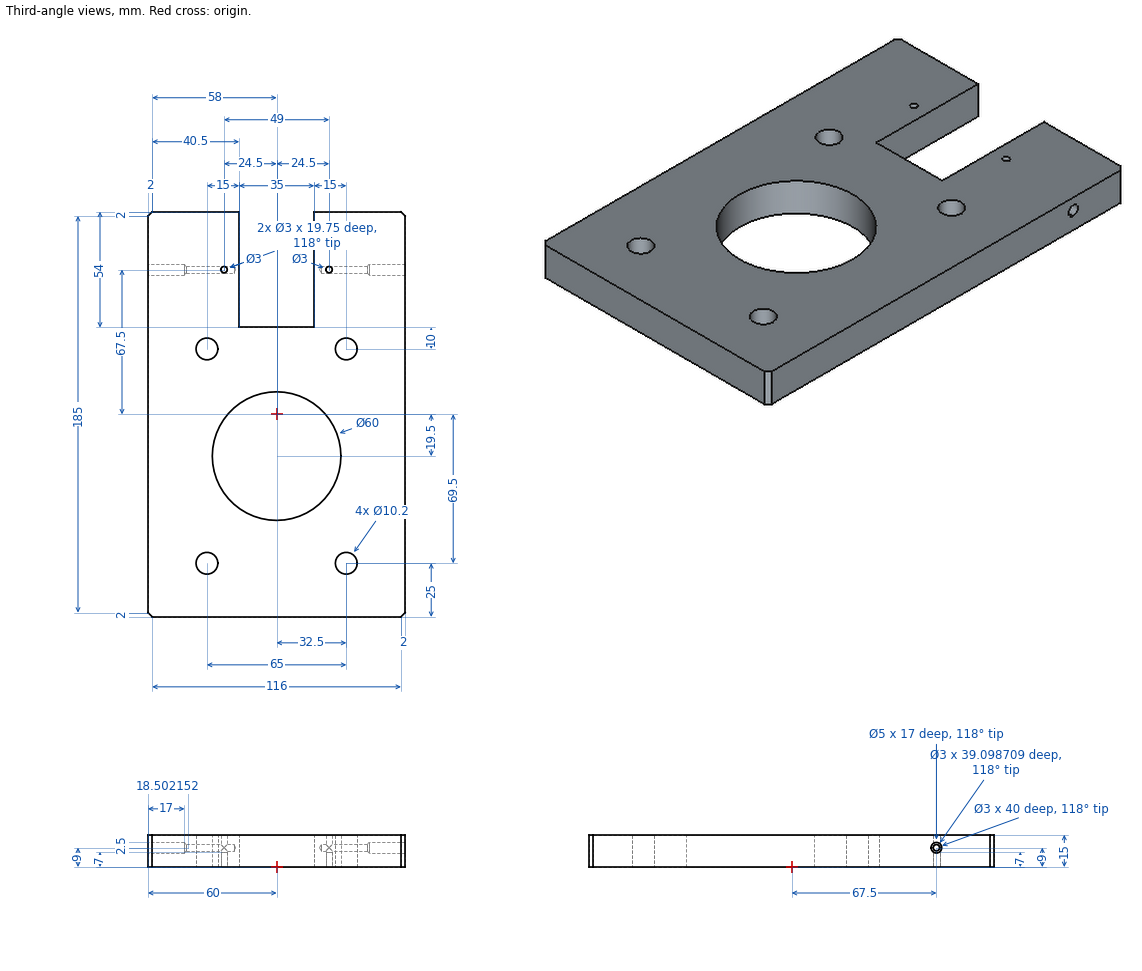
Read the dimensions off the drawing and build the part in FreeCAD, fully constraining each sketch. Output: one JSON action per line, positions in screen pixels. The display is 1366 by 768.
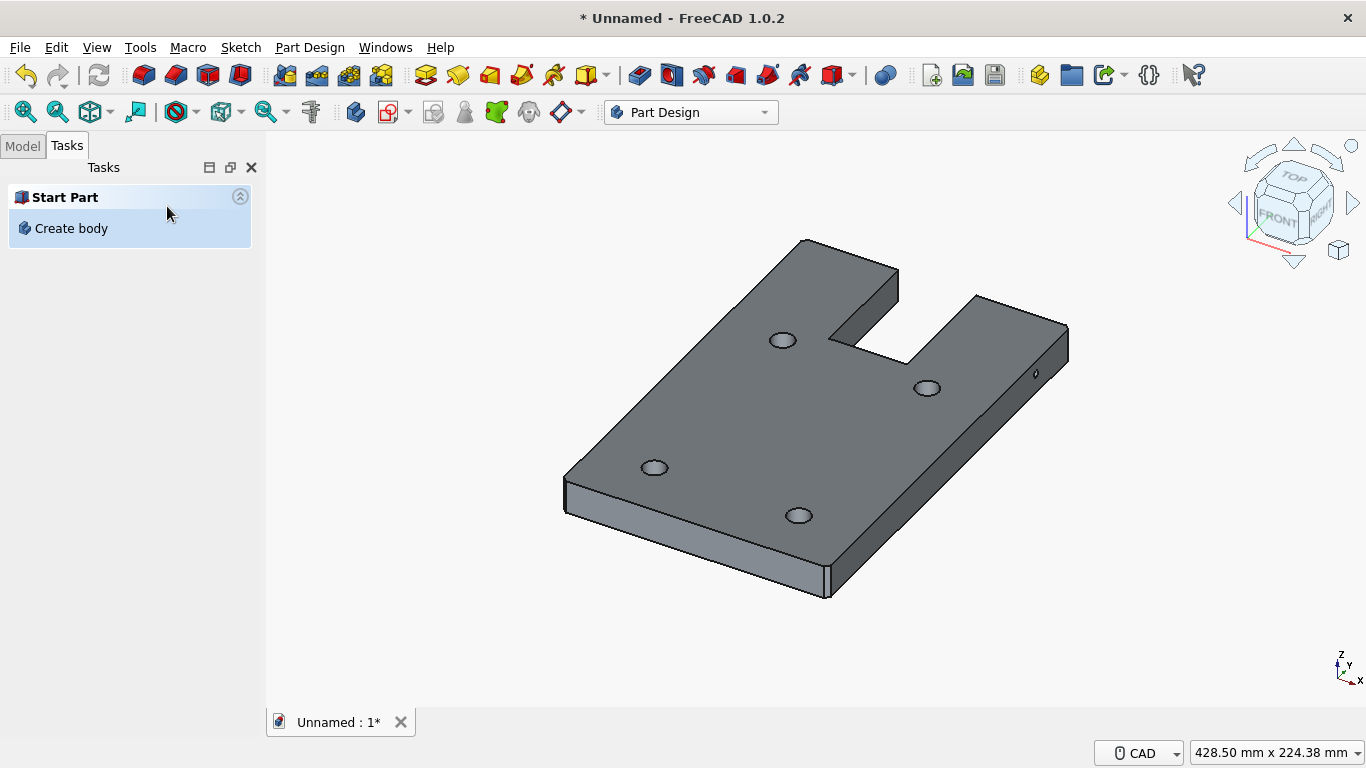
{"action": "key", "text": "6"}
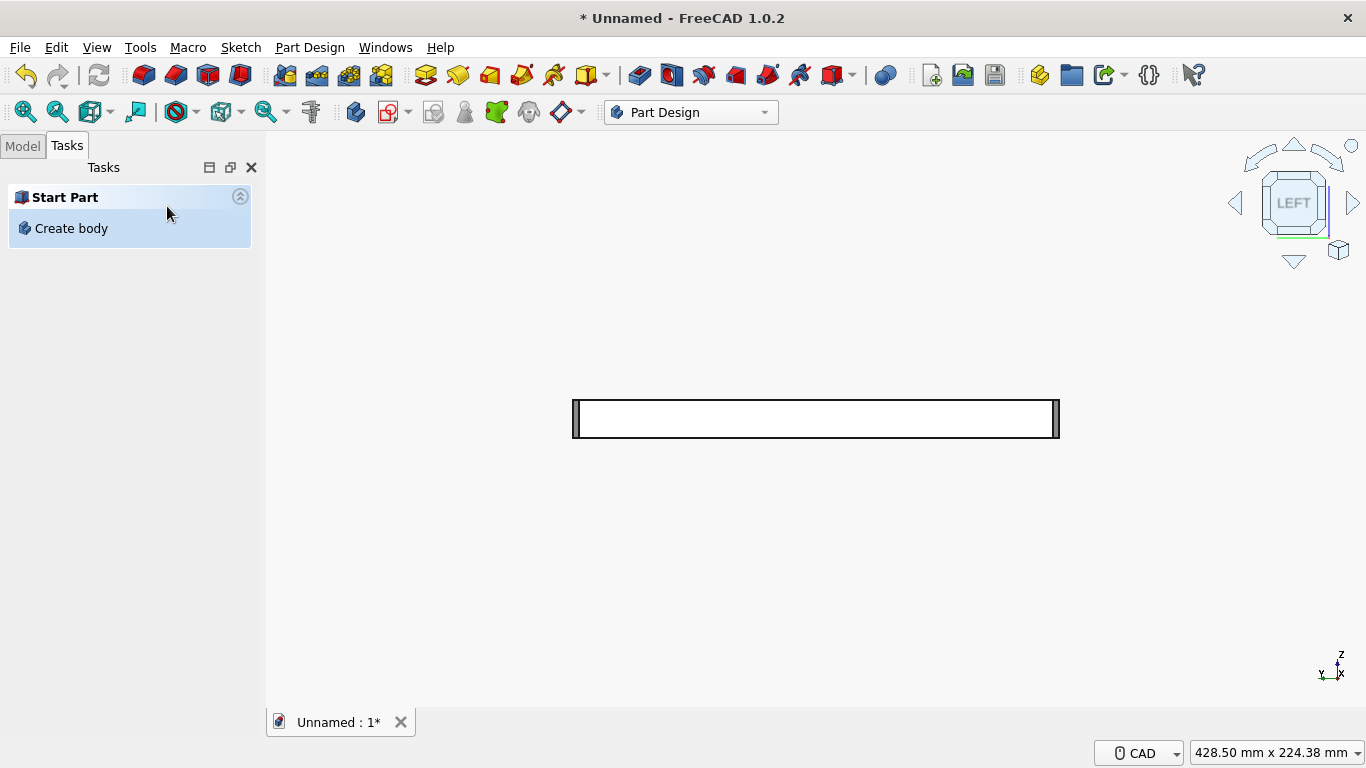
{"action": "key", "text": "v f"}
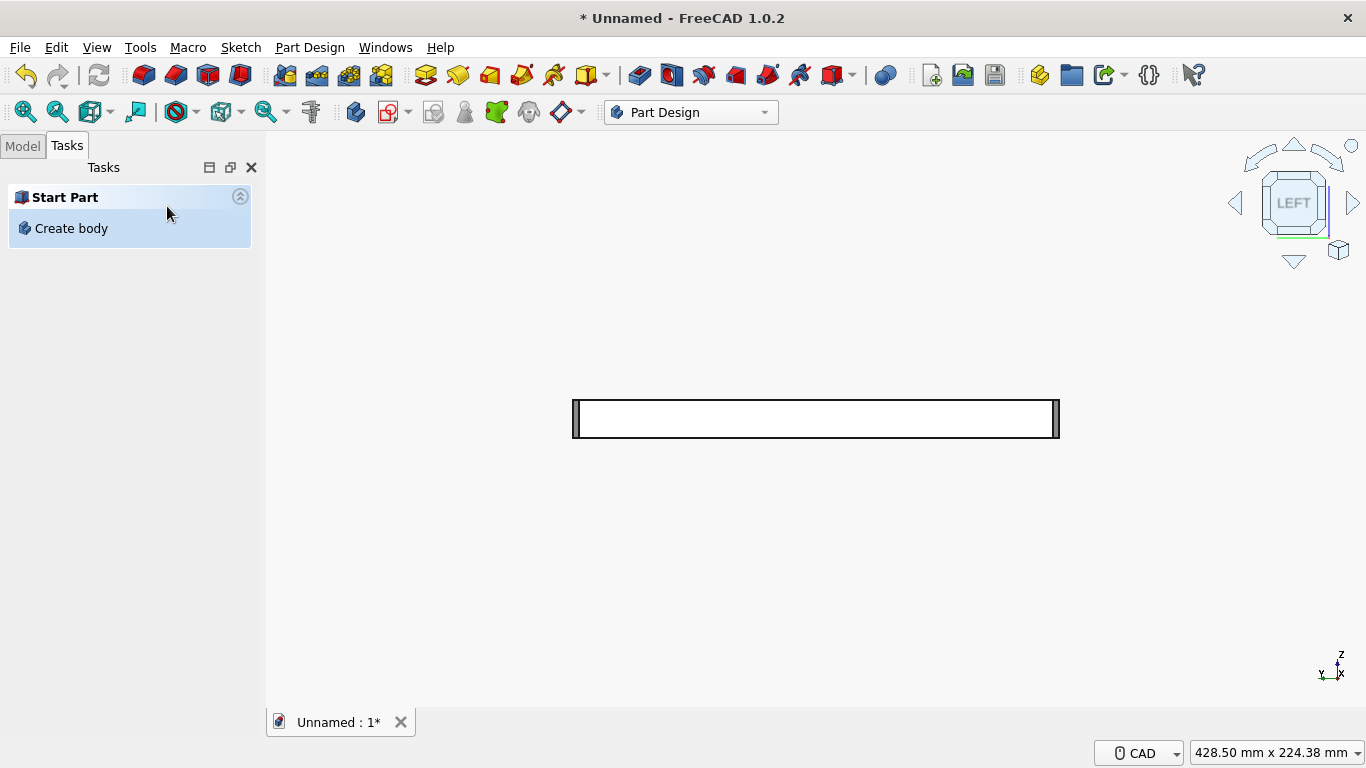
{"action": "left_click", "coordinate": [612, 418]}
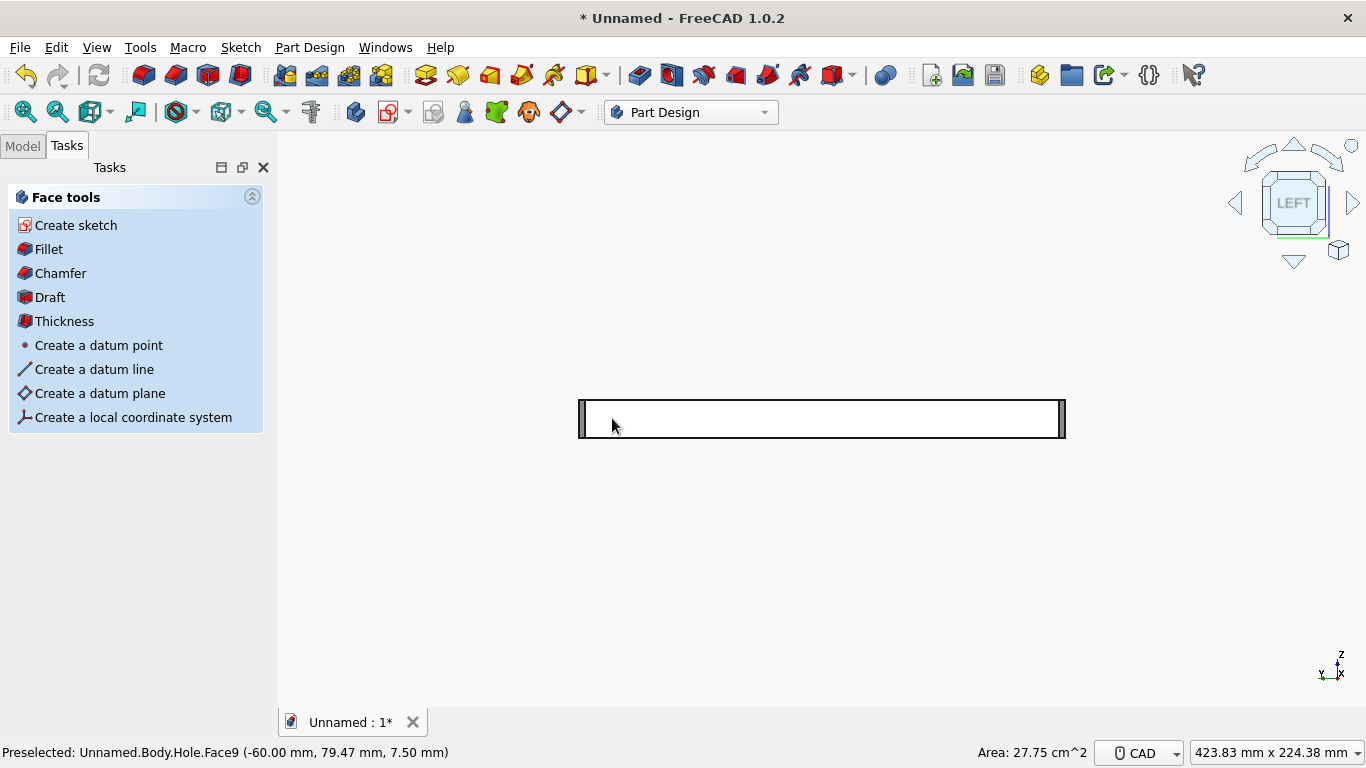
{"action": "left_click", "coordinate": [388, 112]}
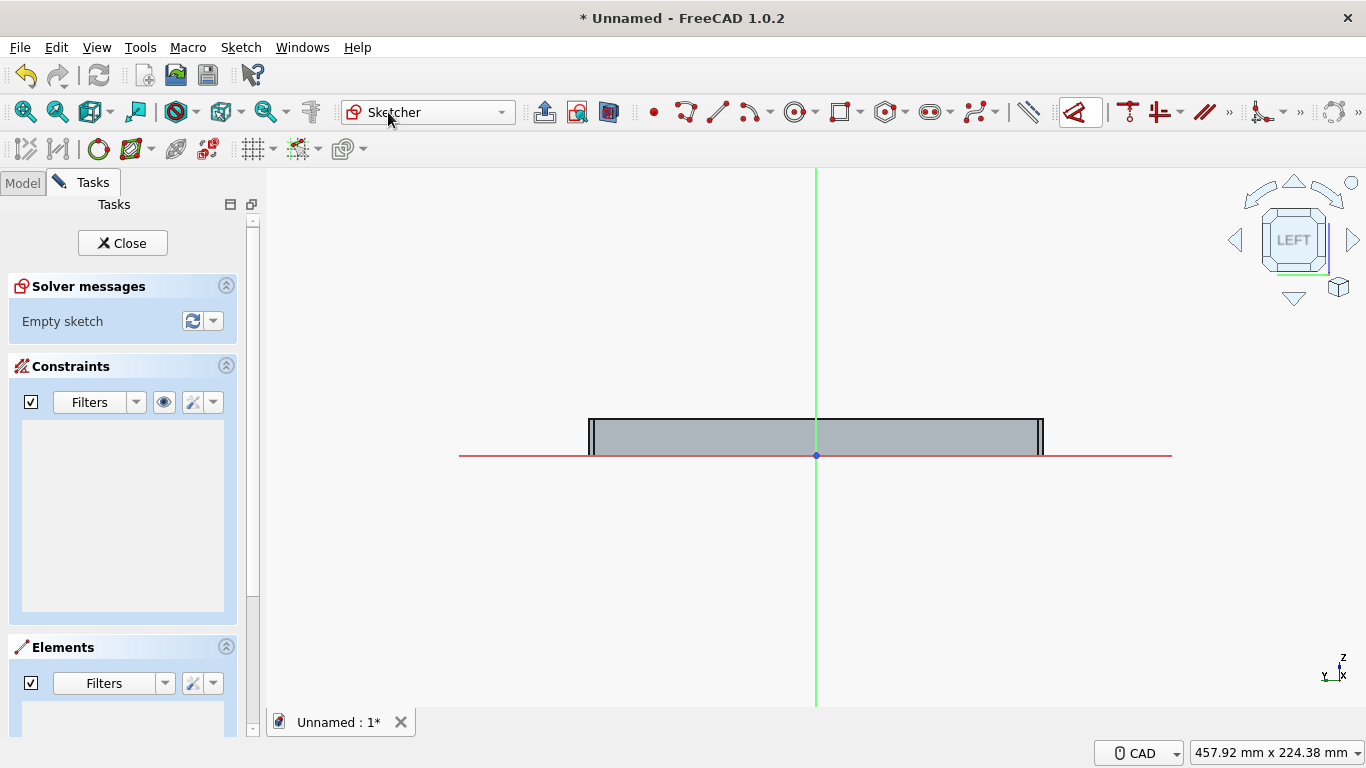
{"action": "scroll", "coordinate": [649, 434], "scroll_direction": "up", "scroll_amount": 15}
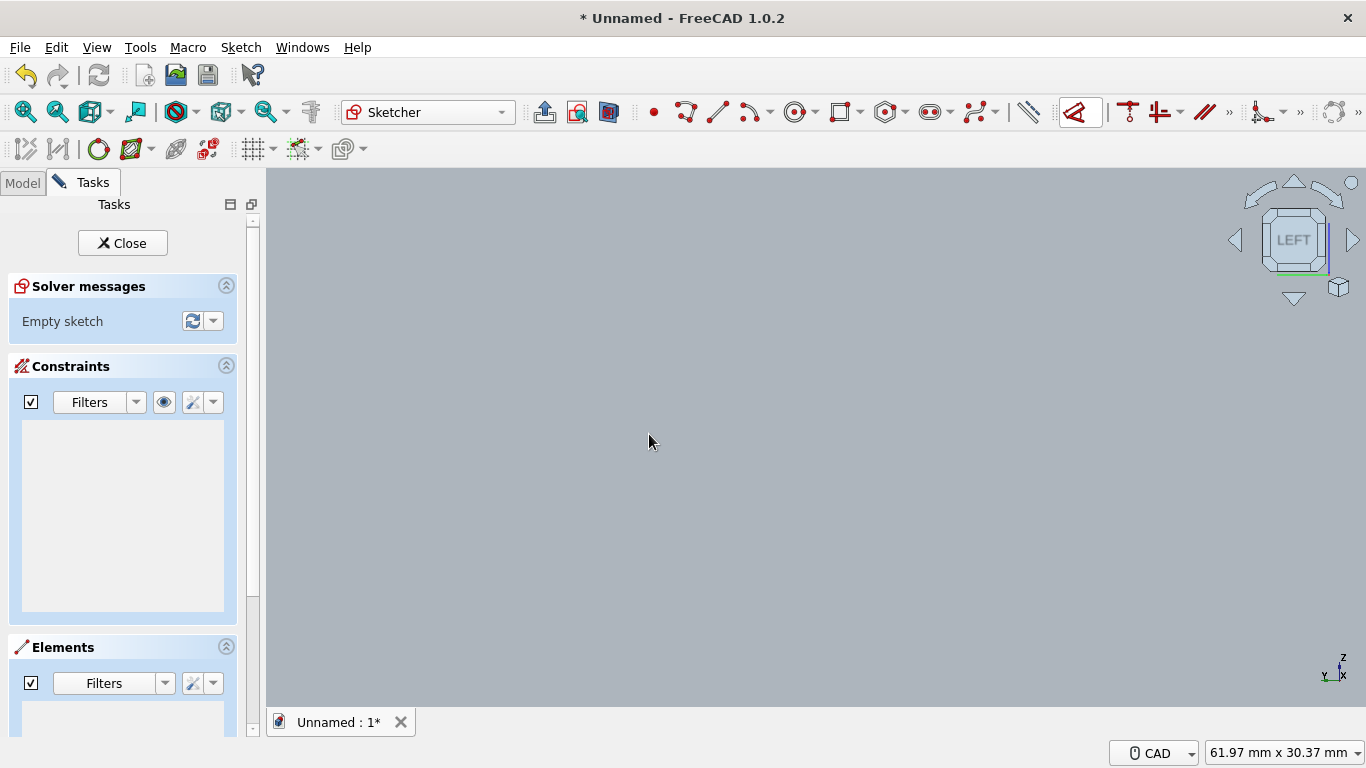
{"action": "scroll", "coordinate": [734, 410], "scroll_direction": "up", "scroll_amount": 4}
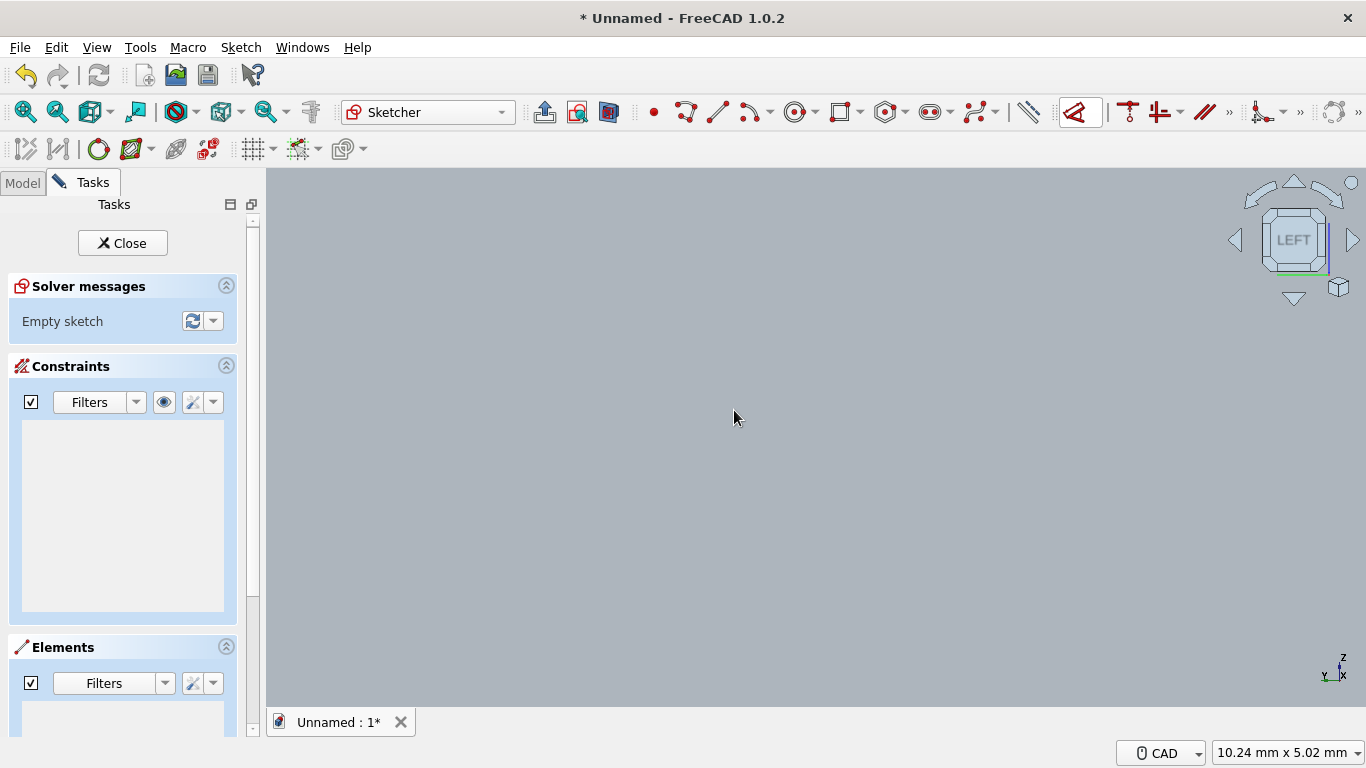
{"action": "left_click", "coordinate": [796, 112]}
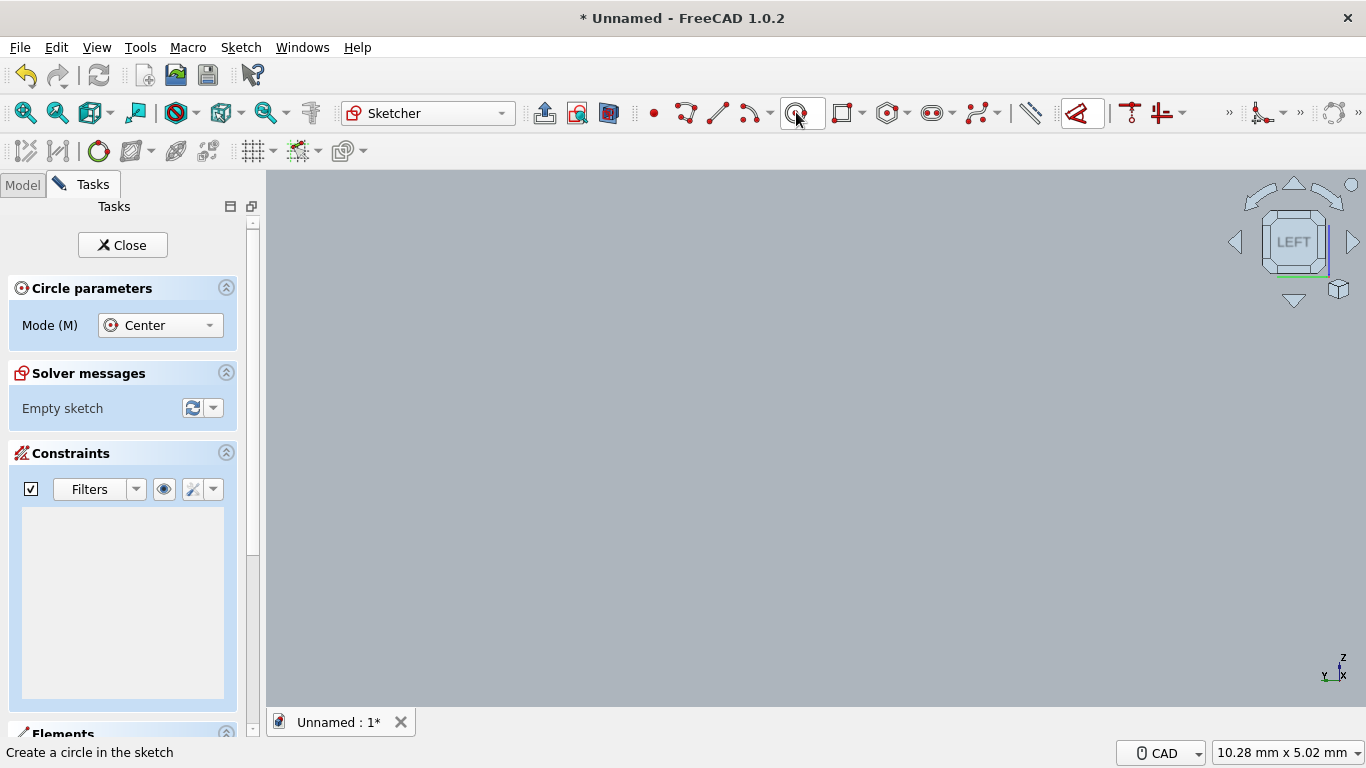
{"action": "left_click", "coordinate": [747, 438]}
{"action": "mouse_move", "coordinate": [860, 325]}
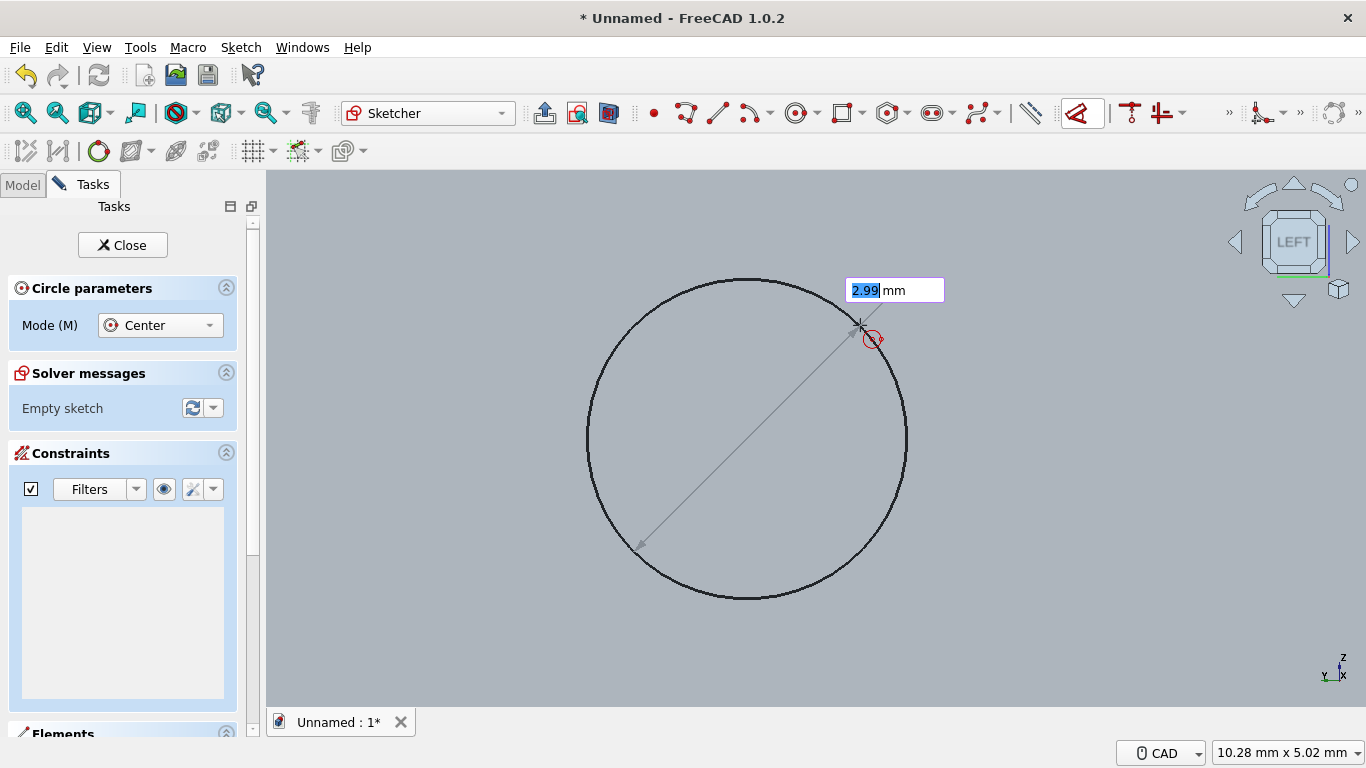
{"action": "type", "text": "3"}
{"action": "key", "text": "Return"}
{"action": "key", "text": "Escape"}